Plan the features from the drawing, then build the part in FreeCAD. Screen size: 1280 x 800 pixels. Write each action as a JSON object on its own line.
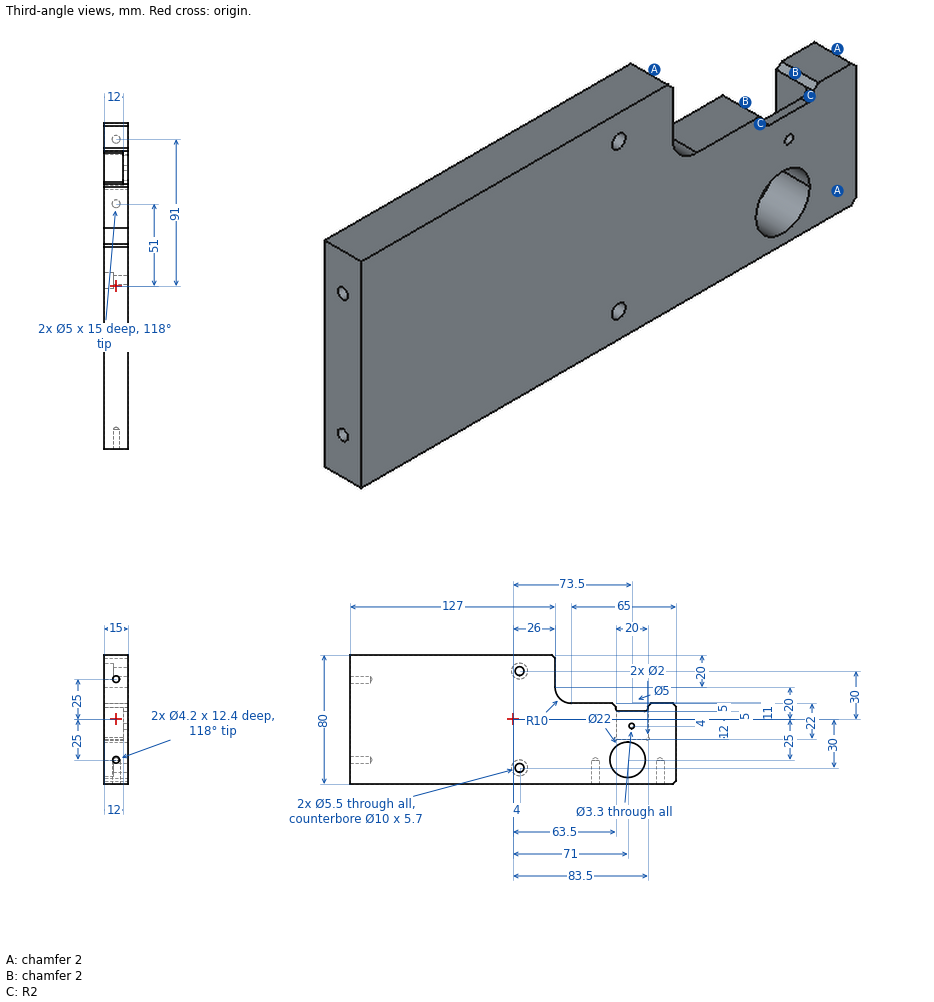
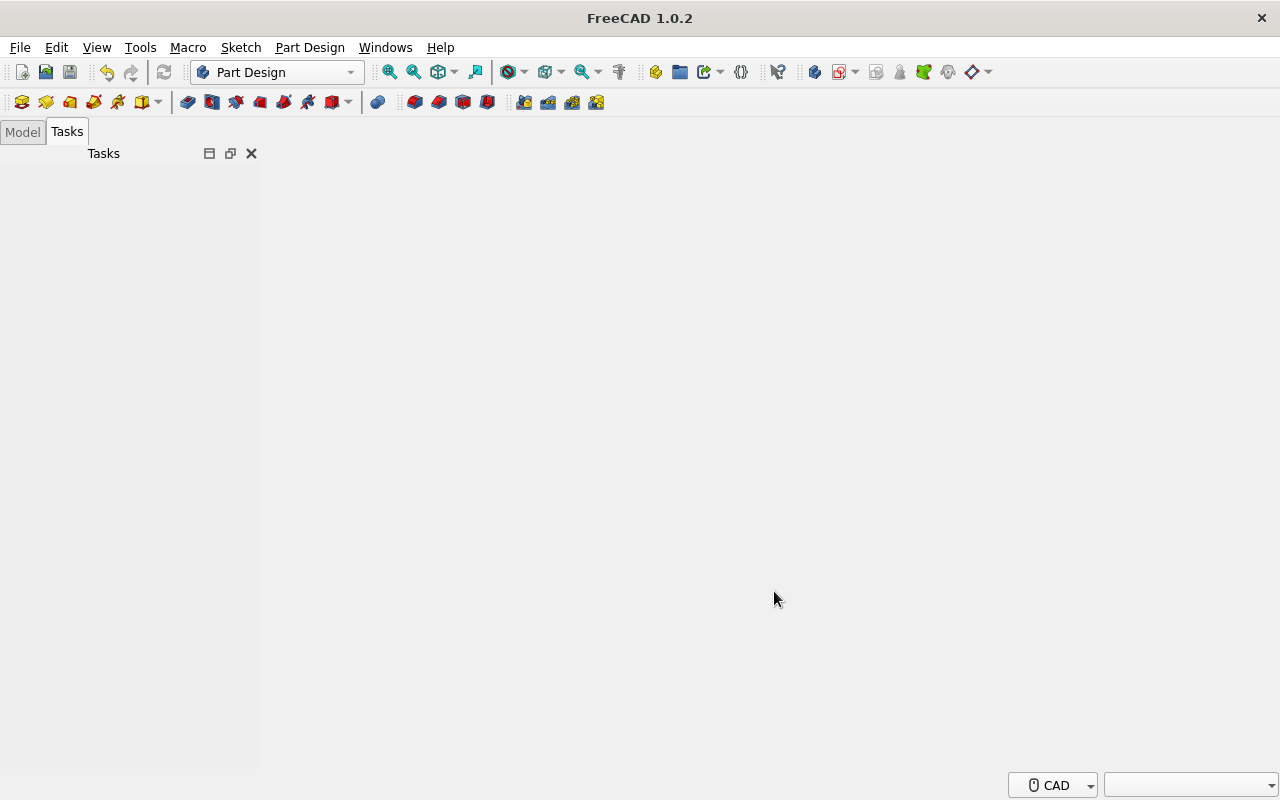
{"action": "left_click", "coordinate": [22, 72]}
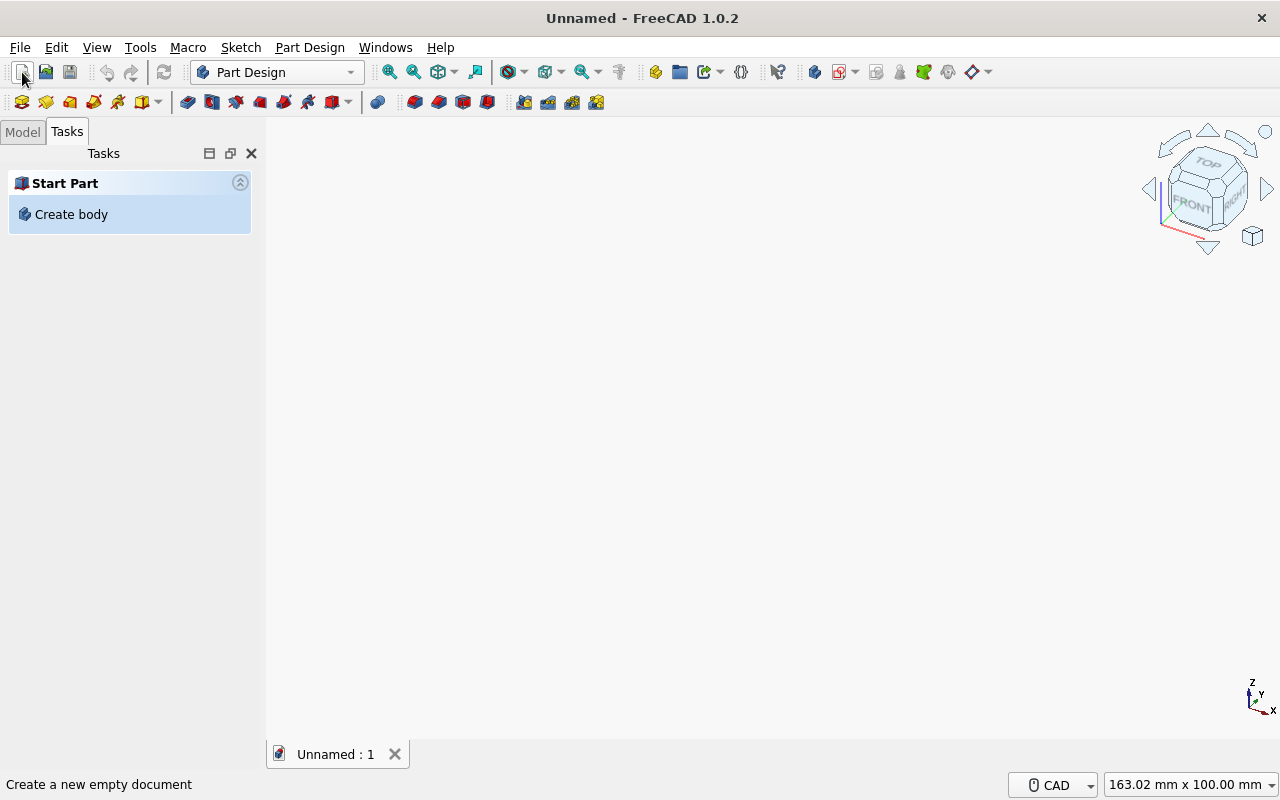
{"action": "left_click", "coordinate": [840, 72]}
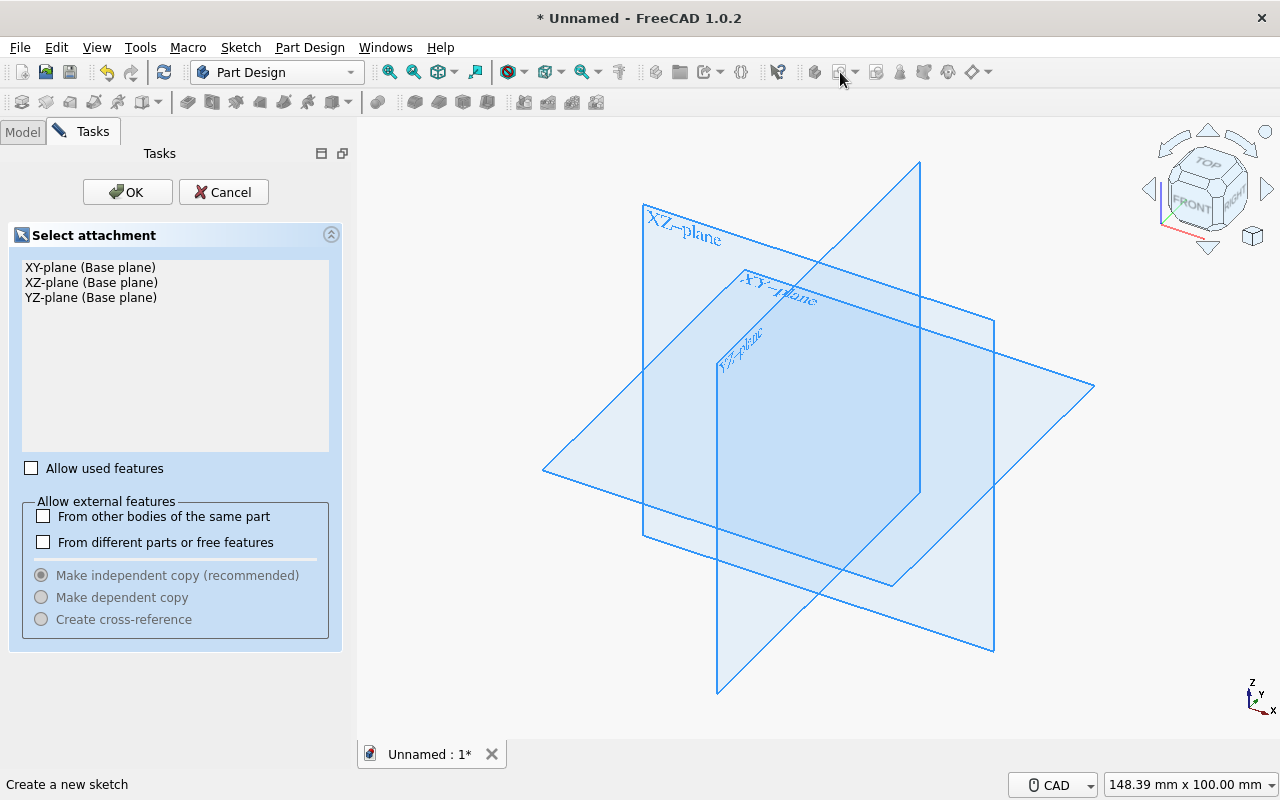
{"action": "left_click", "coordinate": [82, 298]}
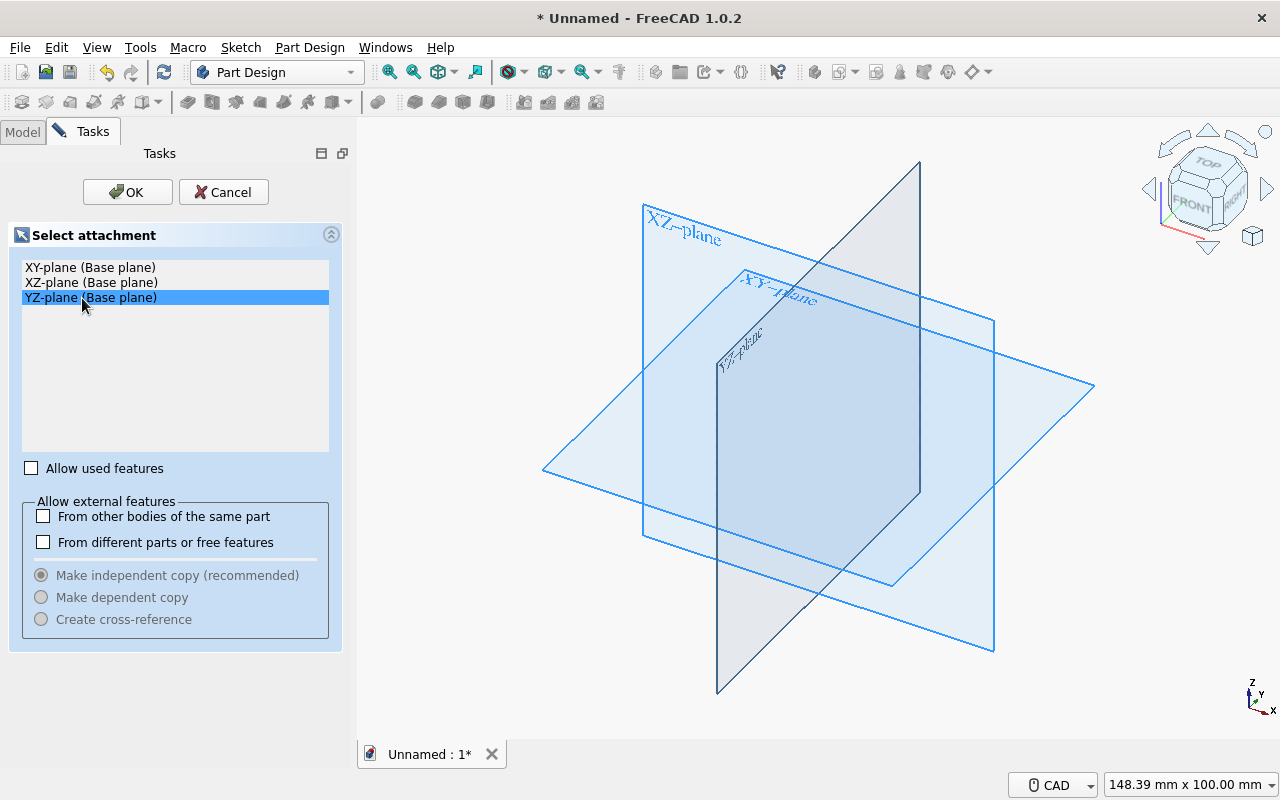
{"action": "left_click", "coordinate": [128, 192]}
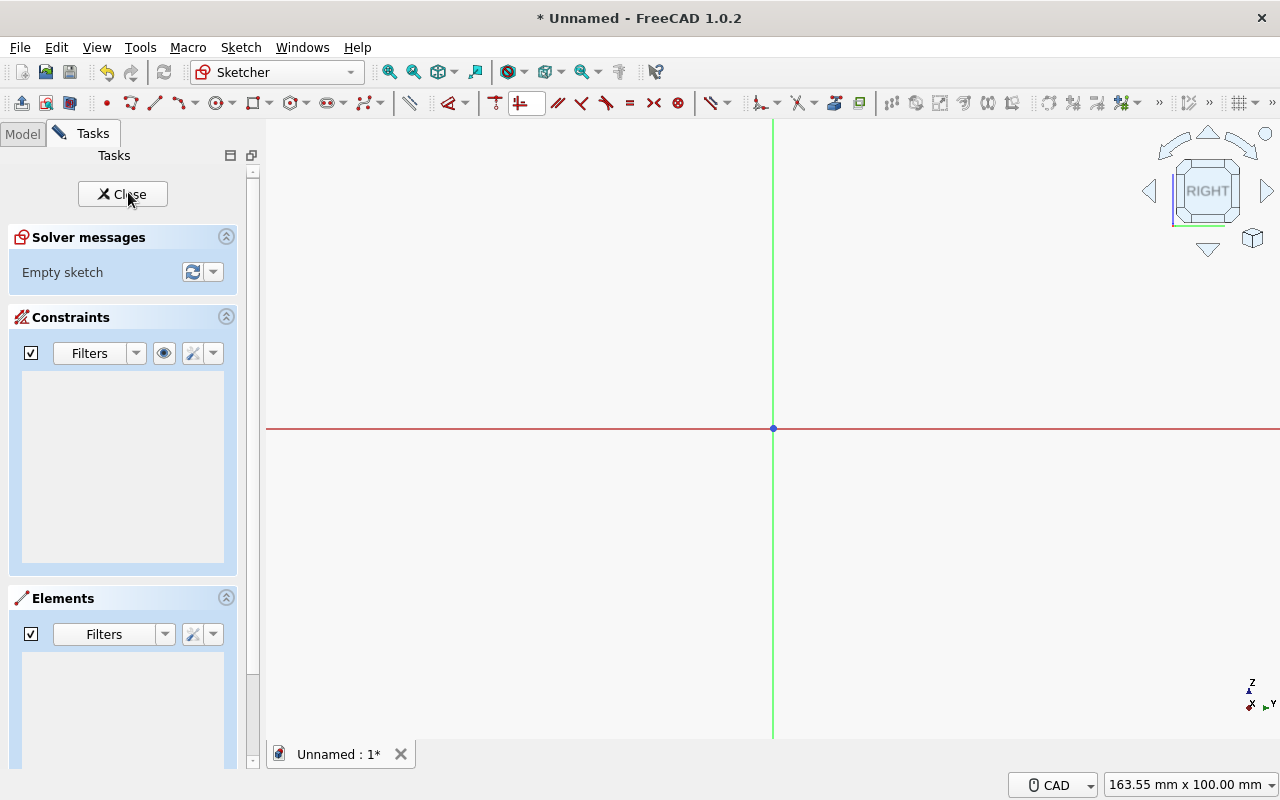
{"action": "scroll", "coordinate": [649, 429], "scroll_direction": "down", "scroll_amount": 4}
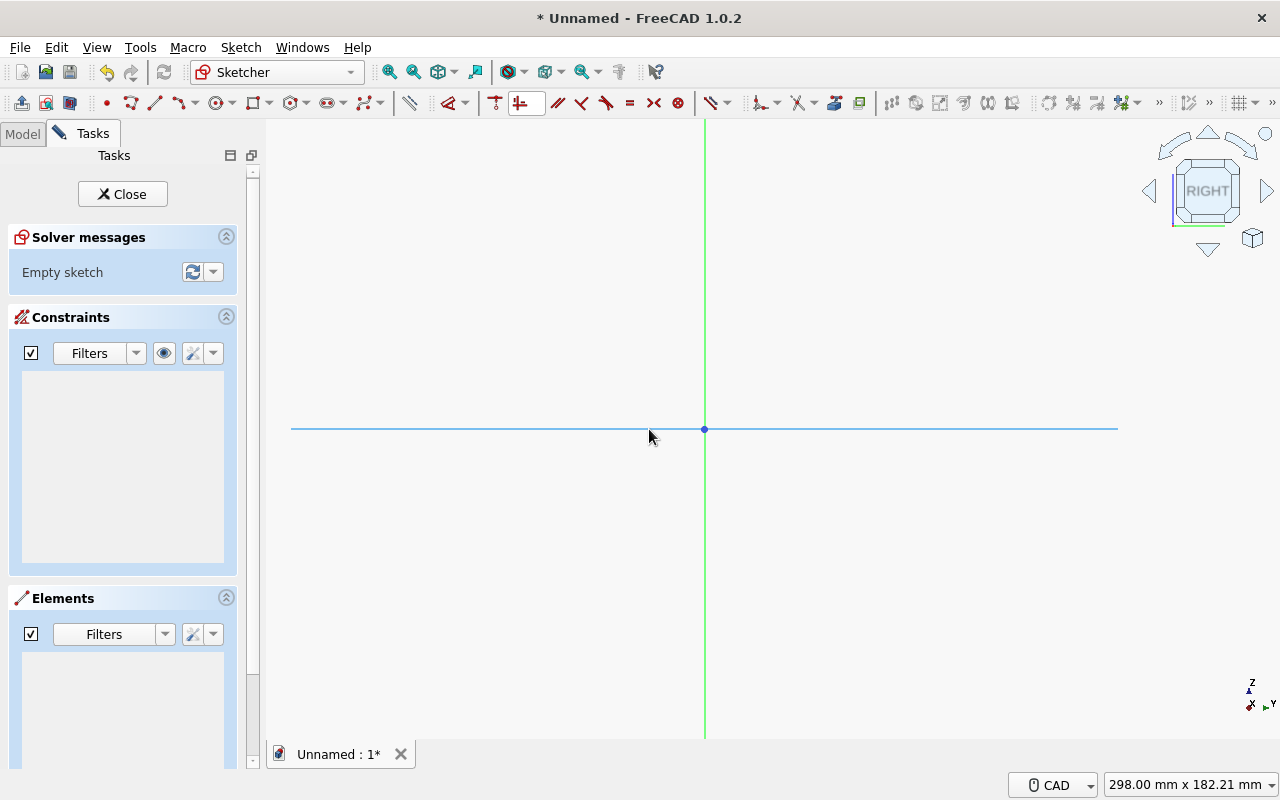
{"action": "left_click", "coordinate": [132, 104]}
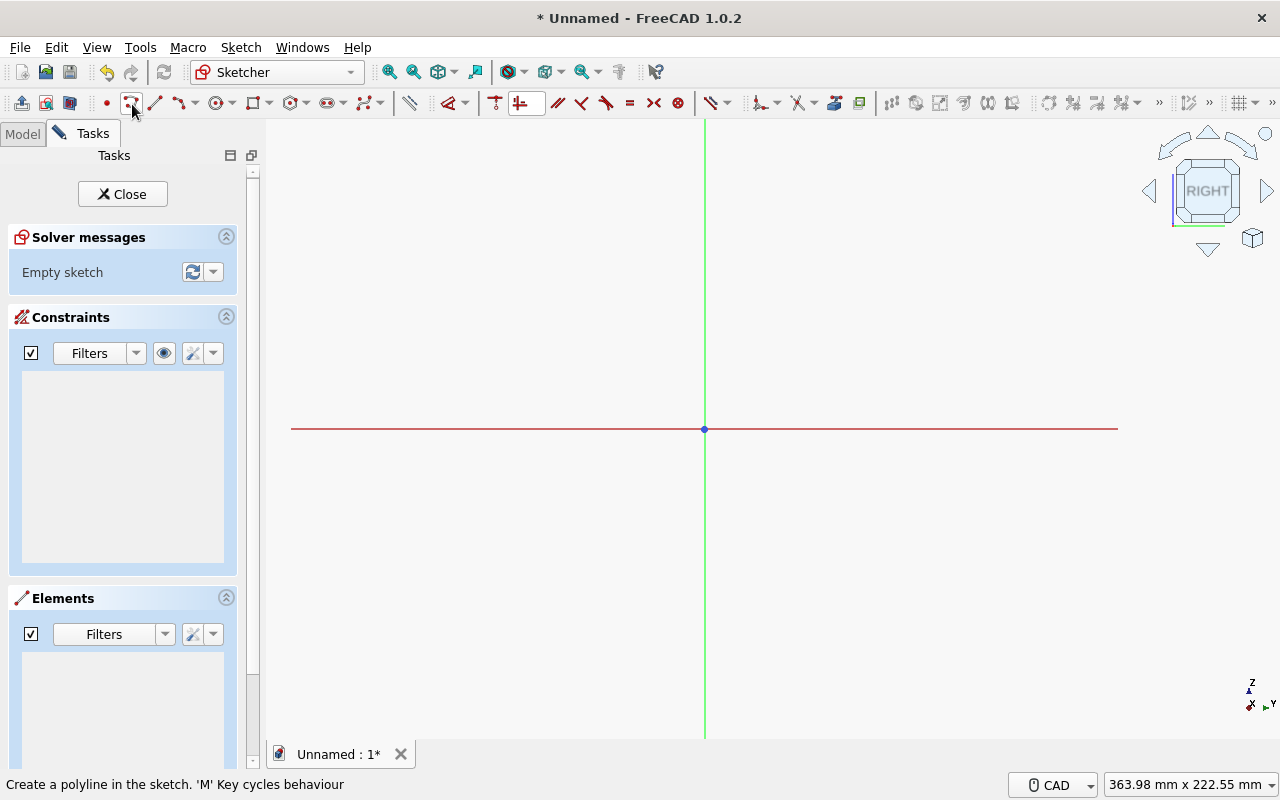
{"action": "left_click", "coordinate": [777, 374]}
{"action": "left_click", "coordinate": [777, 318]}
{"action": "left_click", "coordinate": [424, 318]}
{"action": "left_click", "coordinate": [424, 541]}
{"action": "left_click", "coordinate": [986, 541]}
{"action": "left_click", "coordinate": [986, 401]}
{"action": "left_click", "coordinate": [805, 401]}
{"action": "right_click", "coordinate": [805, 401]}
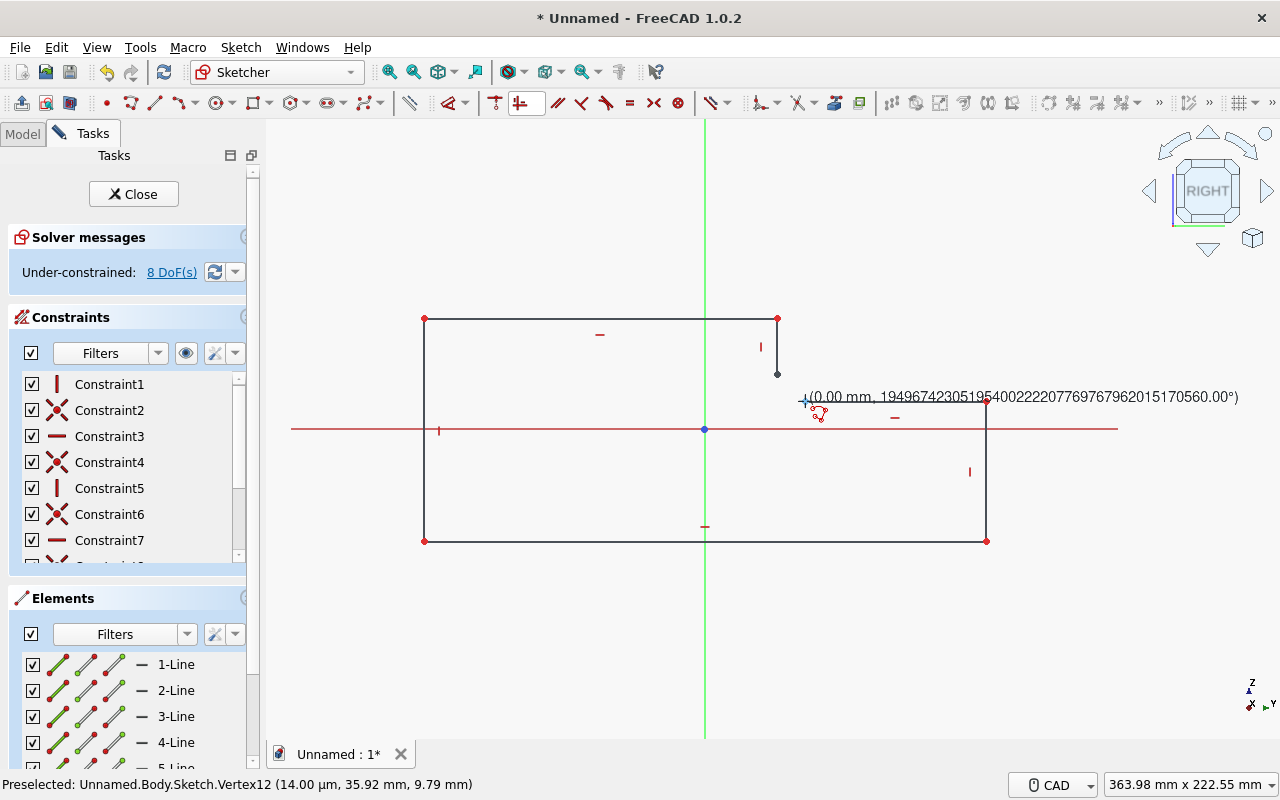
{"action": "left_click", "coordinate": [180, 104]}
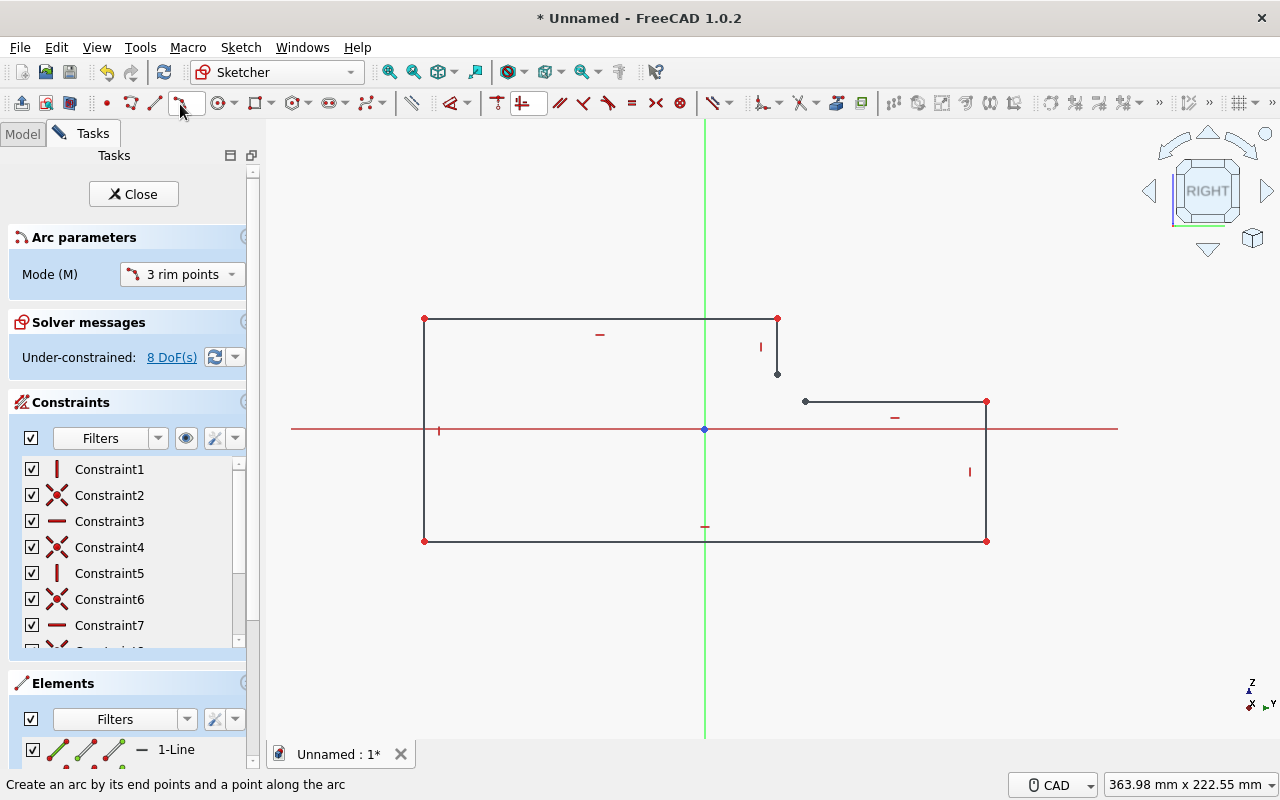
{"action": "left_click", "coordinate": [805, 402]}
{"action": "left_click", "coordinate": [777, 375]}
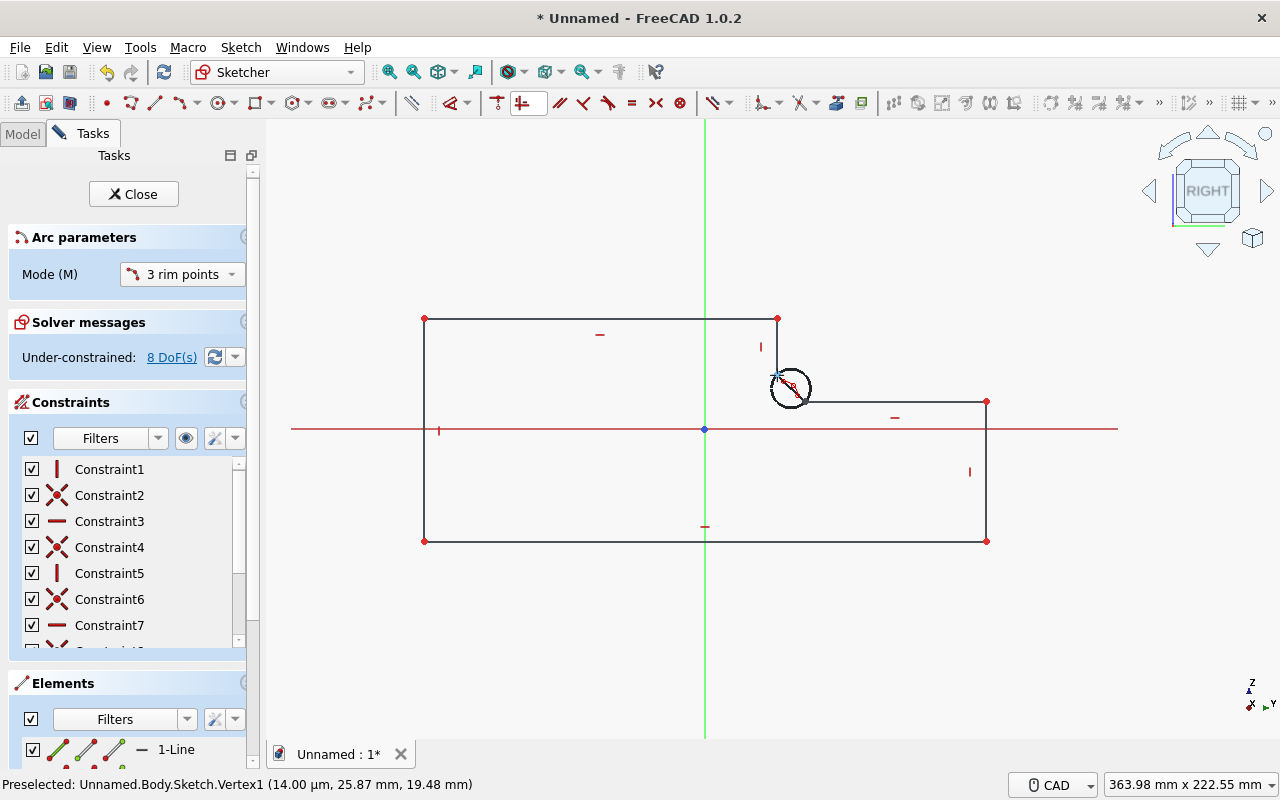
{"action": "scroll", "coordinate": [786, 393], "scroll_direction": "up", "scroll_amount": 4}